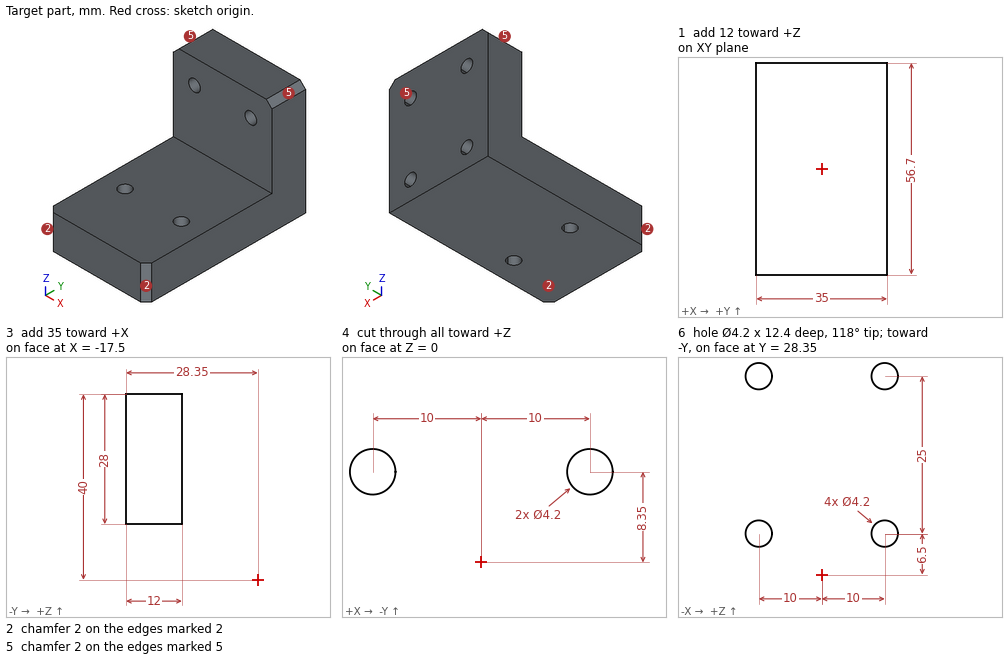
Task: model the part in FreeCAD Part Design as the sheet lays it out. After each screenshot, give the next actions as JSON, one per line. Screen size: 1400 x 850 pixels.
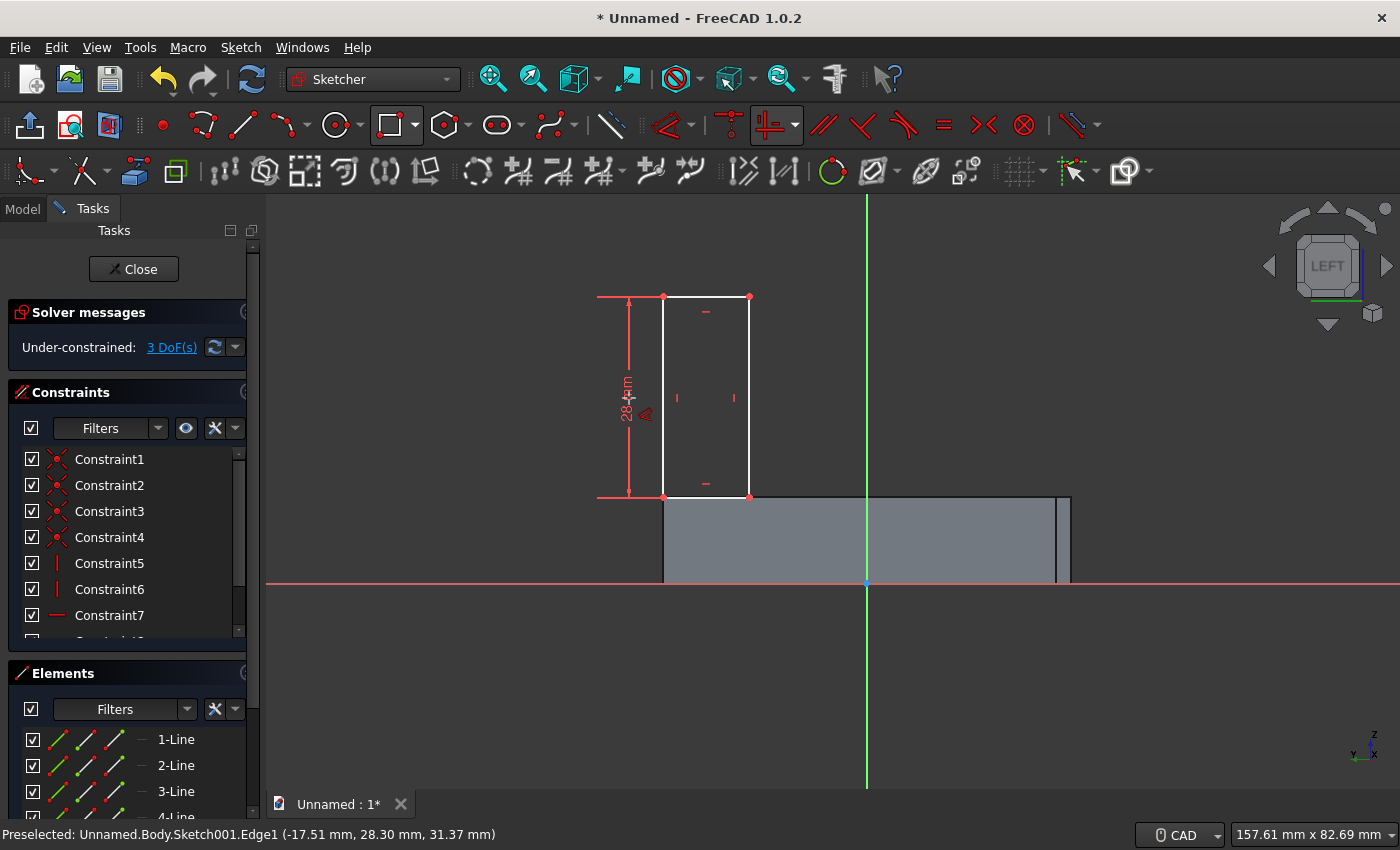
{"action": "left_click", "coordinate": [689, 498]}
{"action": "left_click", "coordinate": [706, 532]}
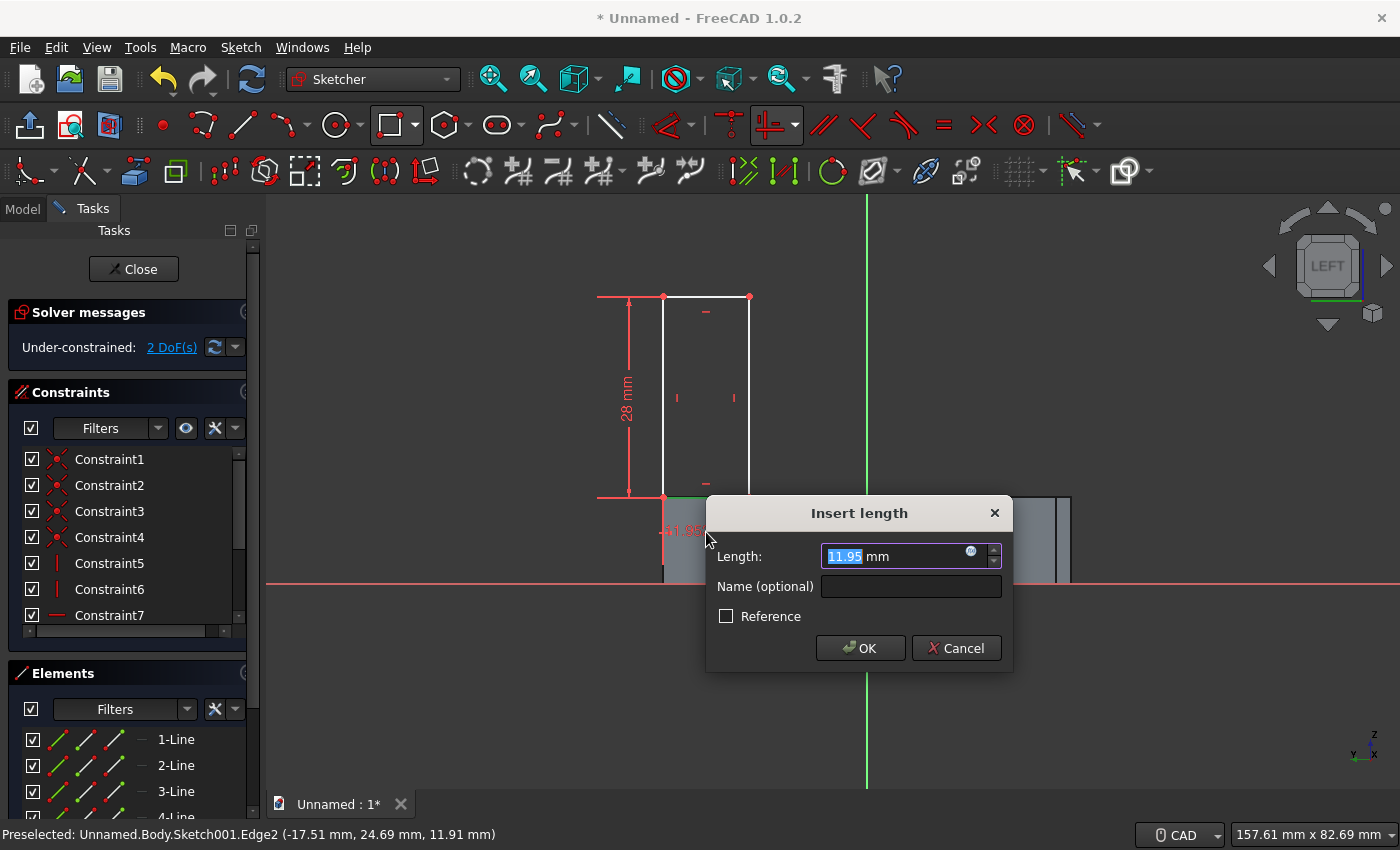
{"action": "type", "text": "12"}
{"action": "key", "text": "Return"}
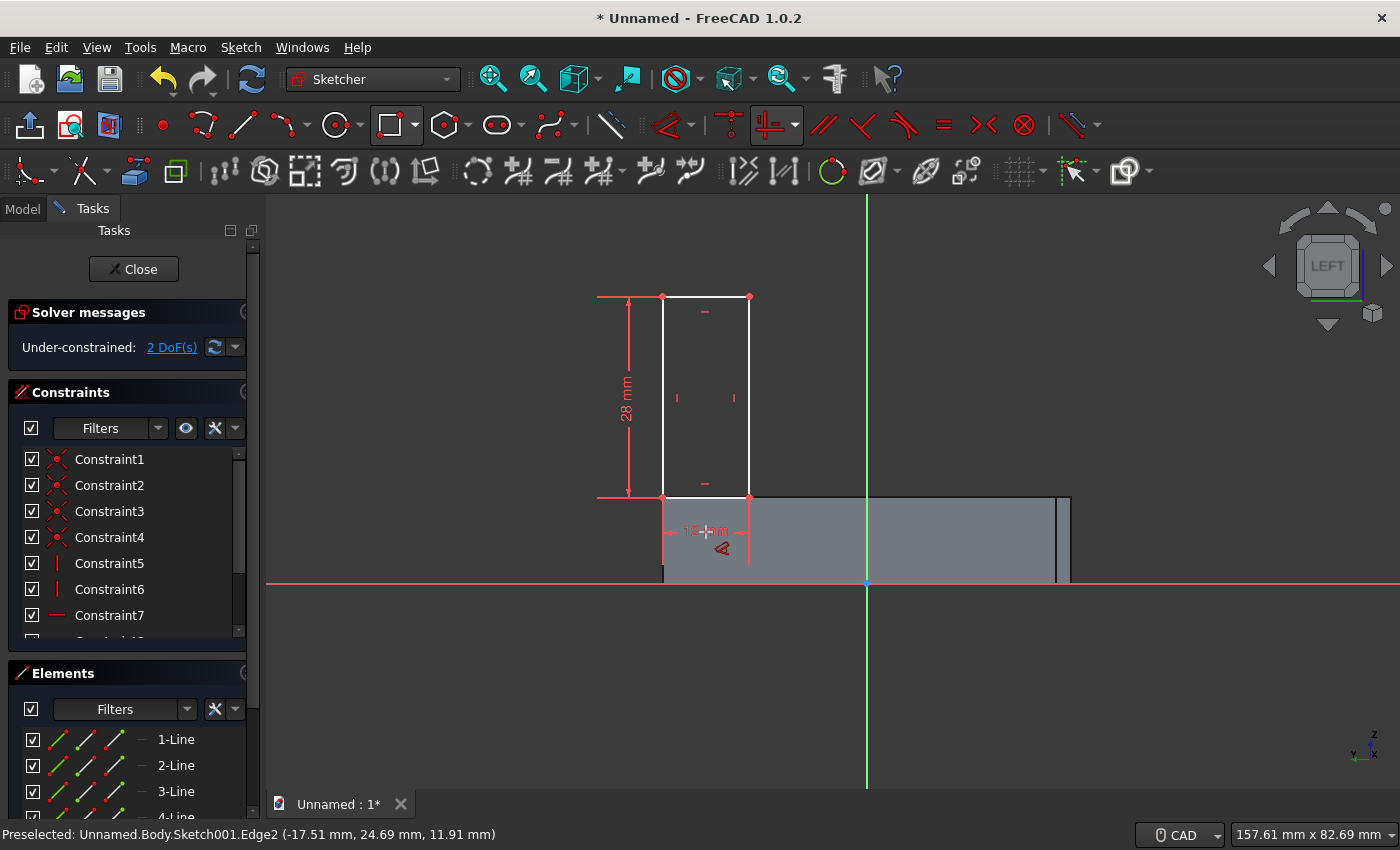
{"action": "left_click", "coordinate": [663, 297]}
{"action": "left_click", "coordinate": [629, 440]}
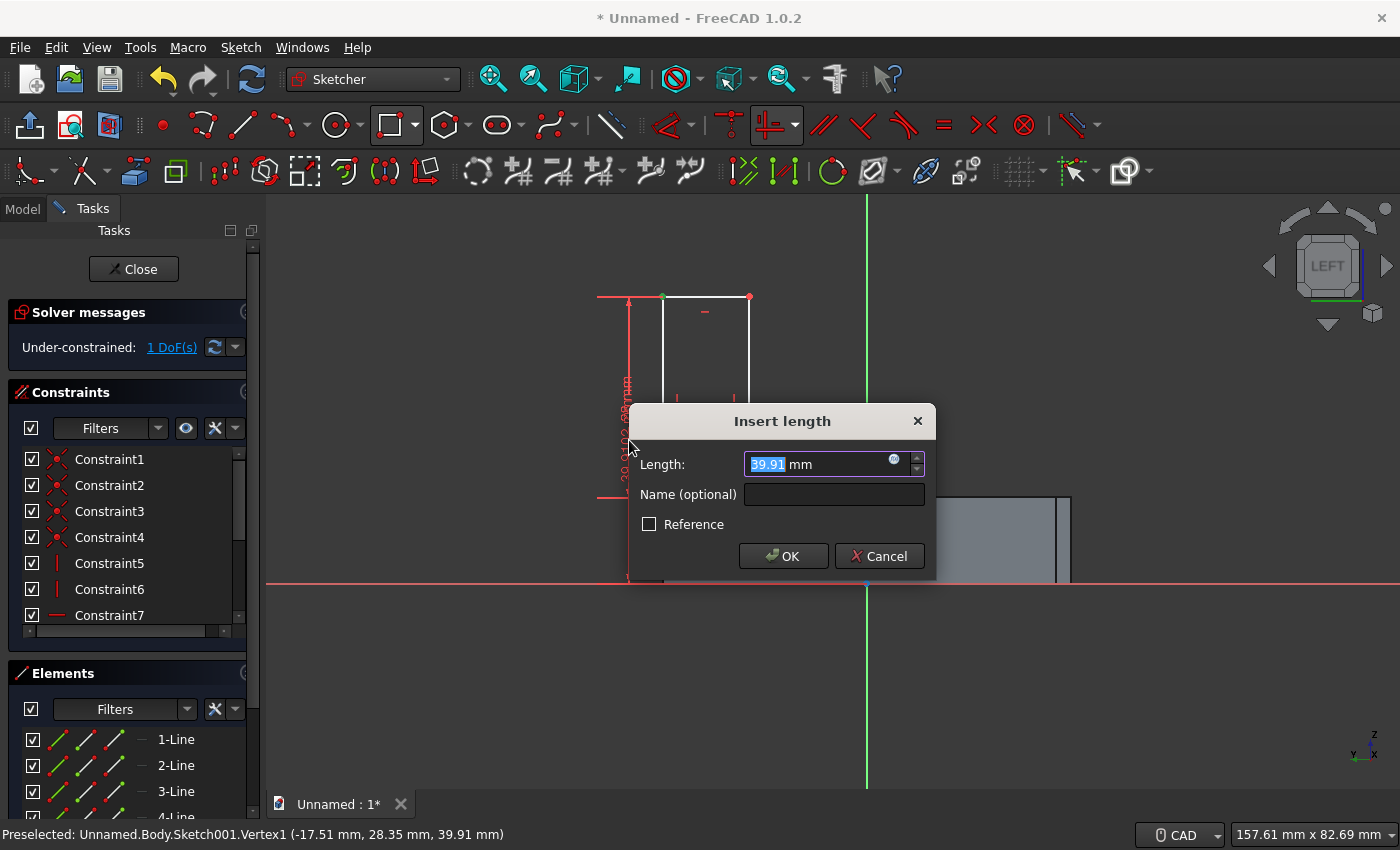
{"action": "type", "text": "40"}
{"action": "key", "text": "Return"}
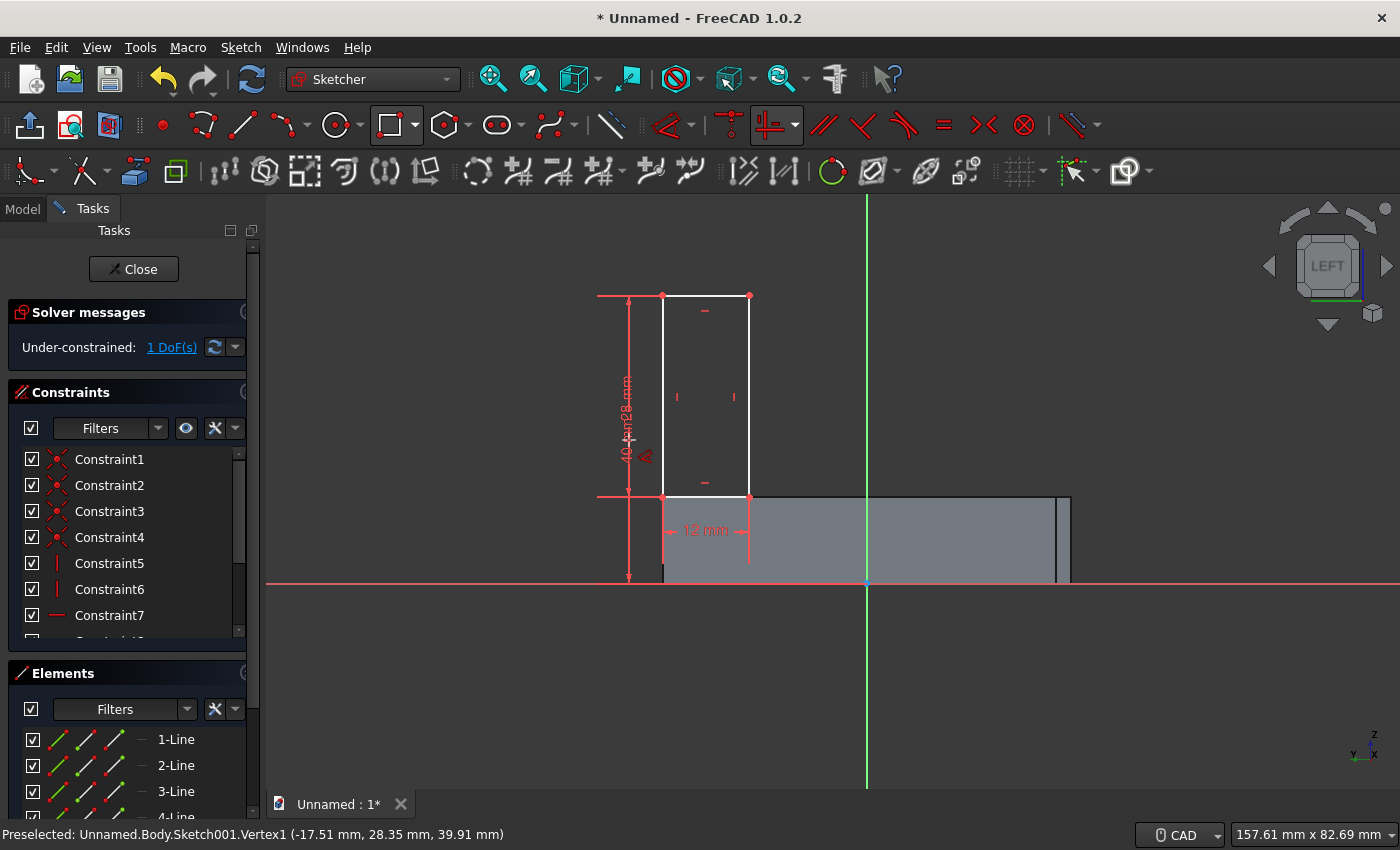
{"action": "left_click", "coordinate": [663, 296]}
{"action": "left_click", "coordinate": [765, 618]}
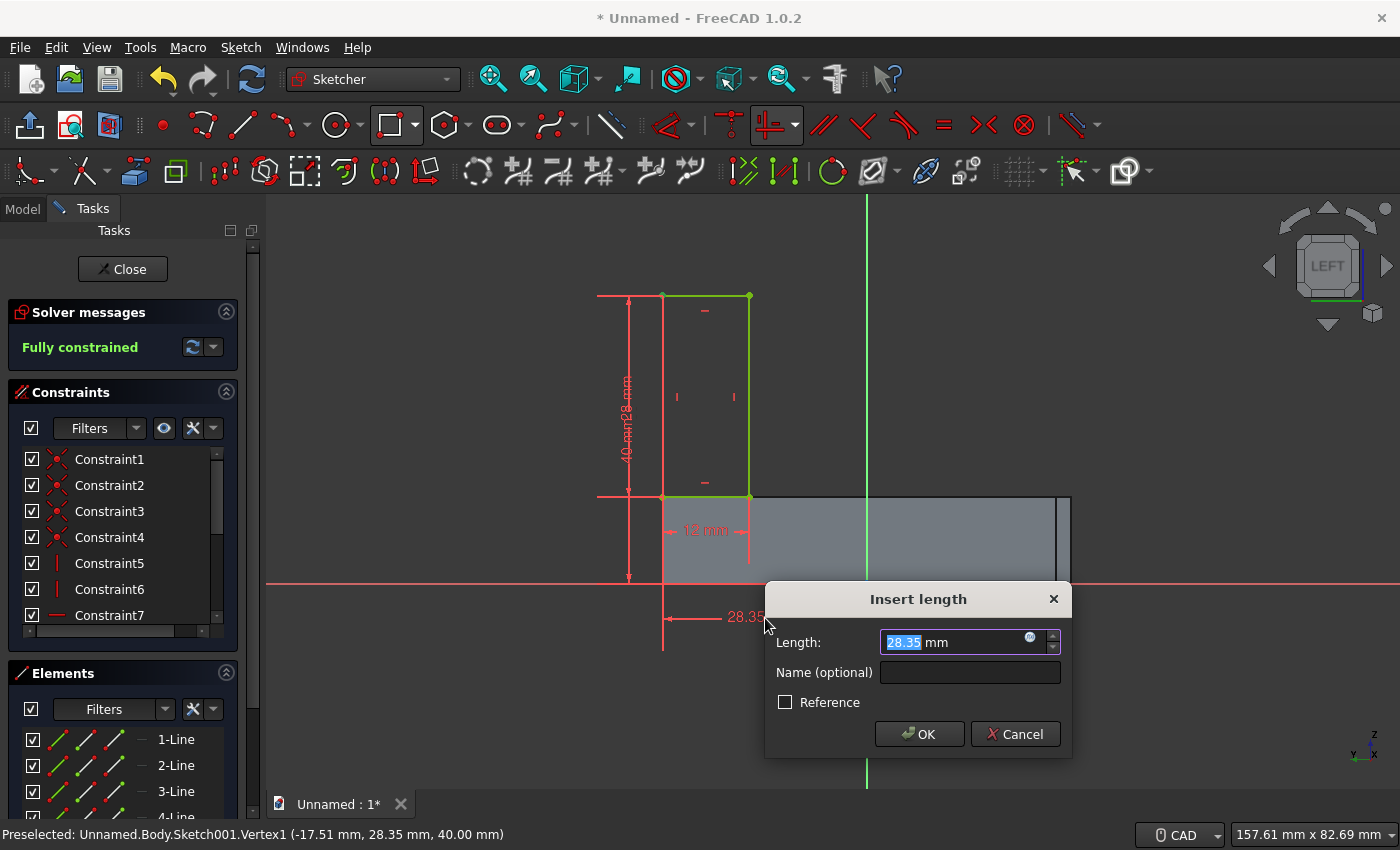
{"action": "type", "text": "28.35"}
{"action": "key", "text": "Return"}
{"action": "key", "text": "Escape"}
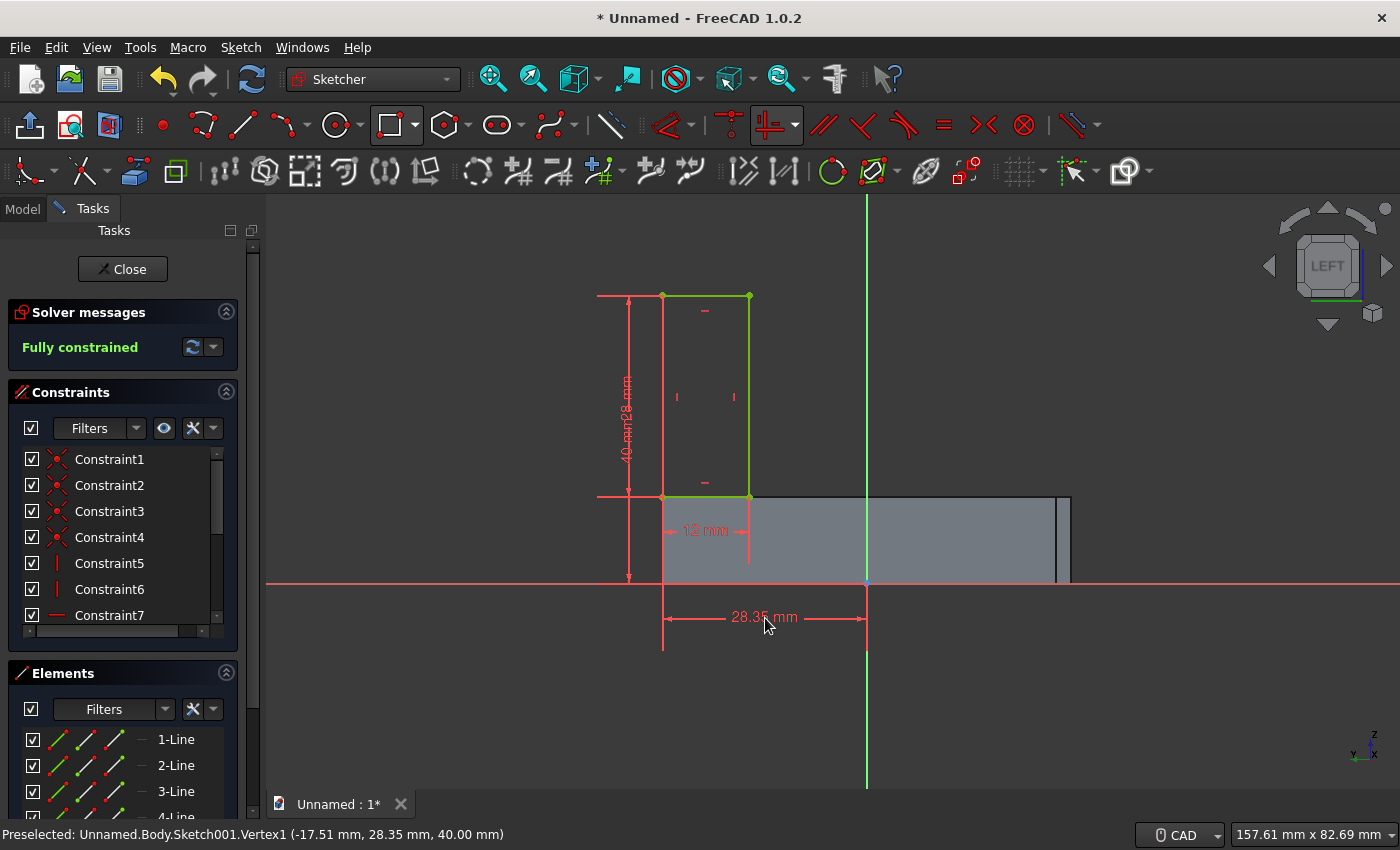
{"action": "left_click", "coordinate": [123, 269]}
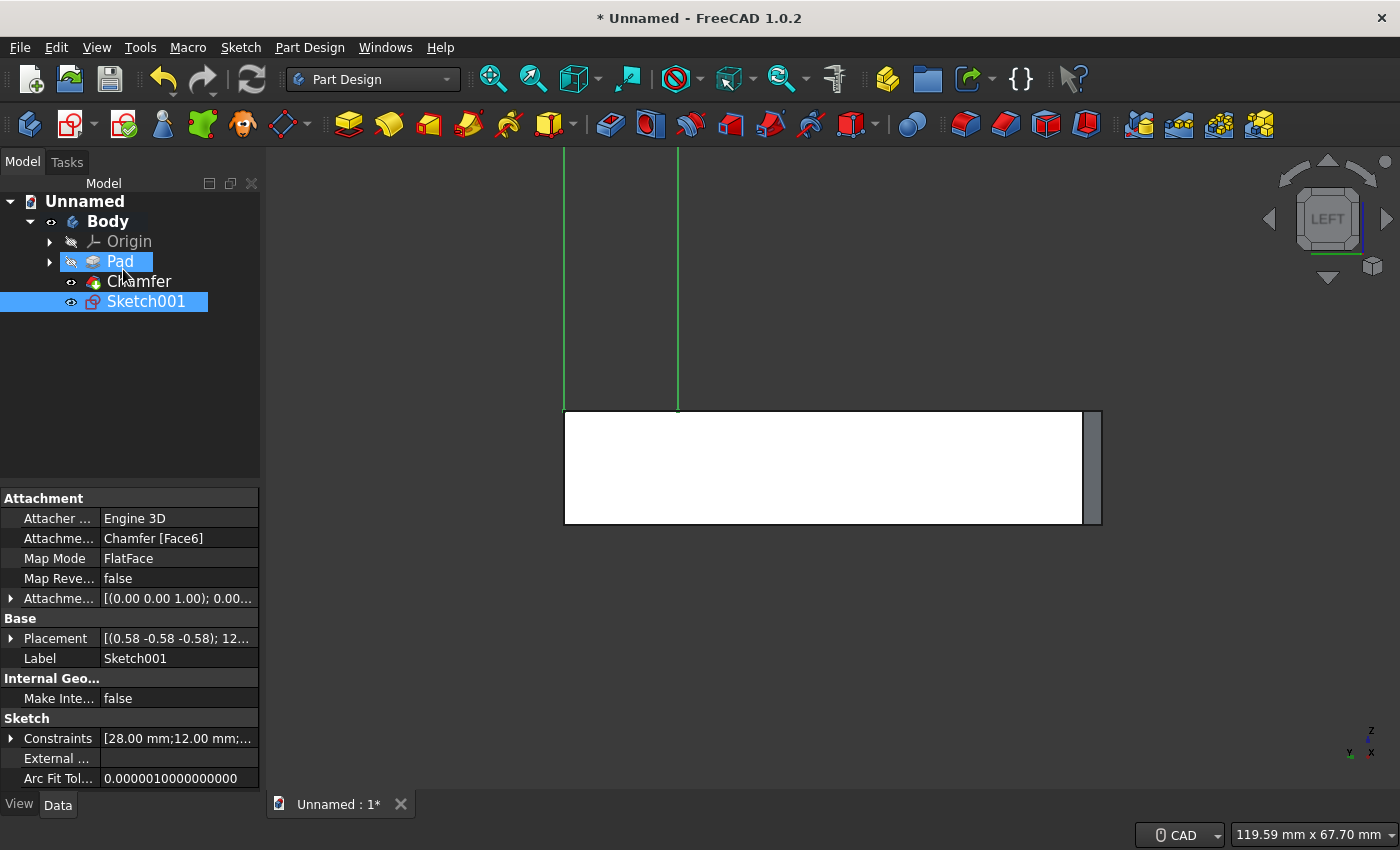
{"action": "left_click", "coordinate": [350, 124]}